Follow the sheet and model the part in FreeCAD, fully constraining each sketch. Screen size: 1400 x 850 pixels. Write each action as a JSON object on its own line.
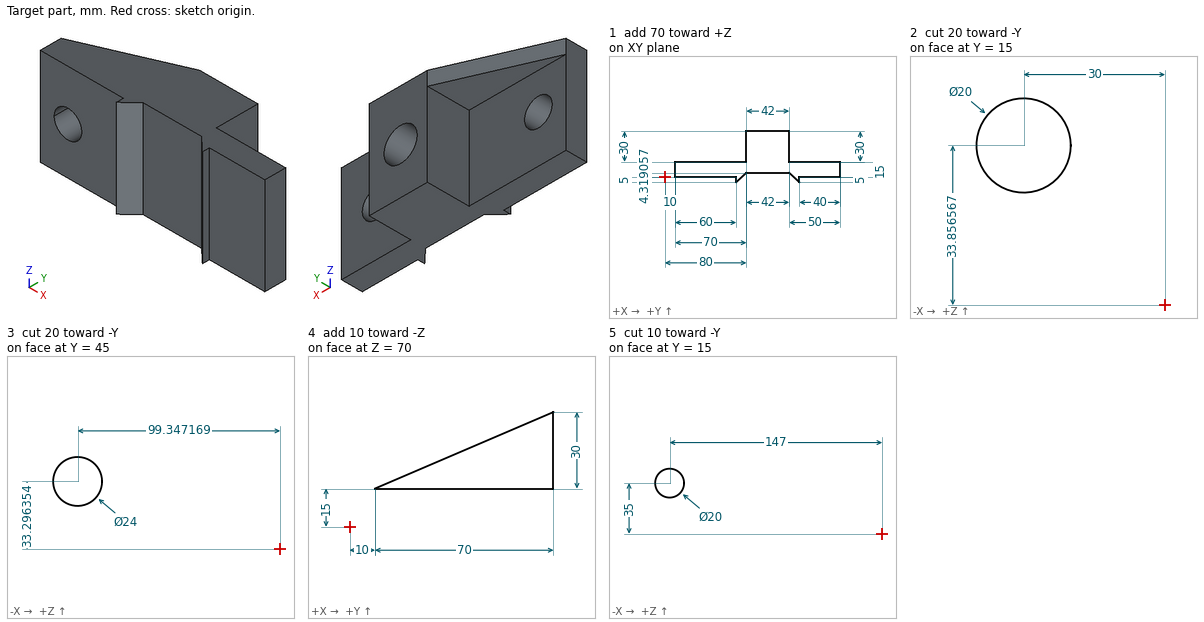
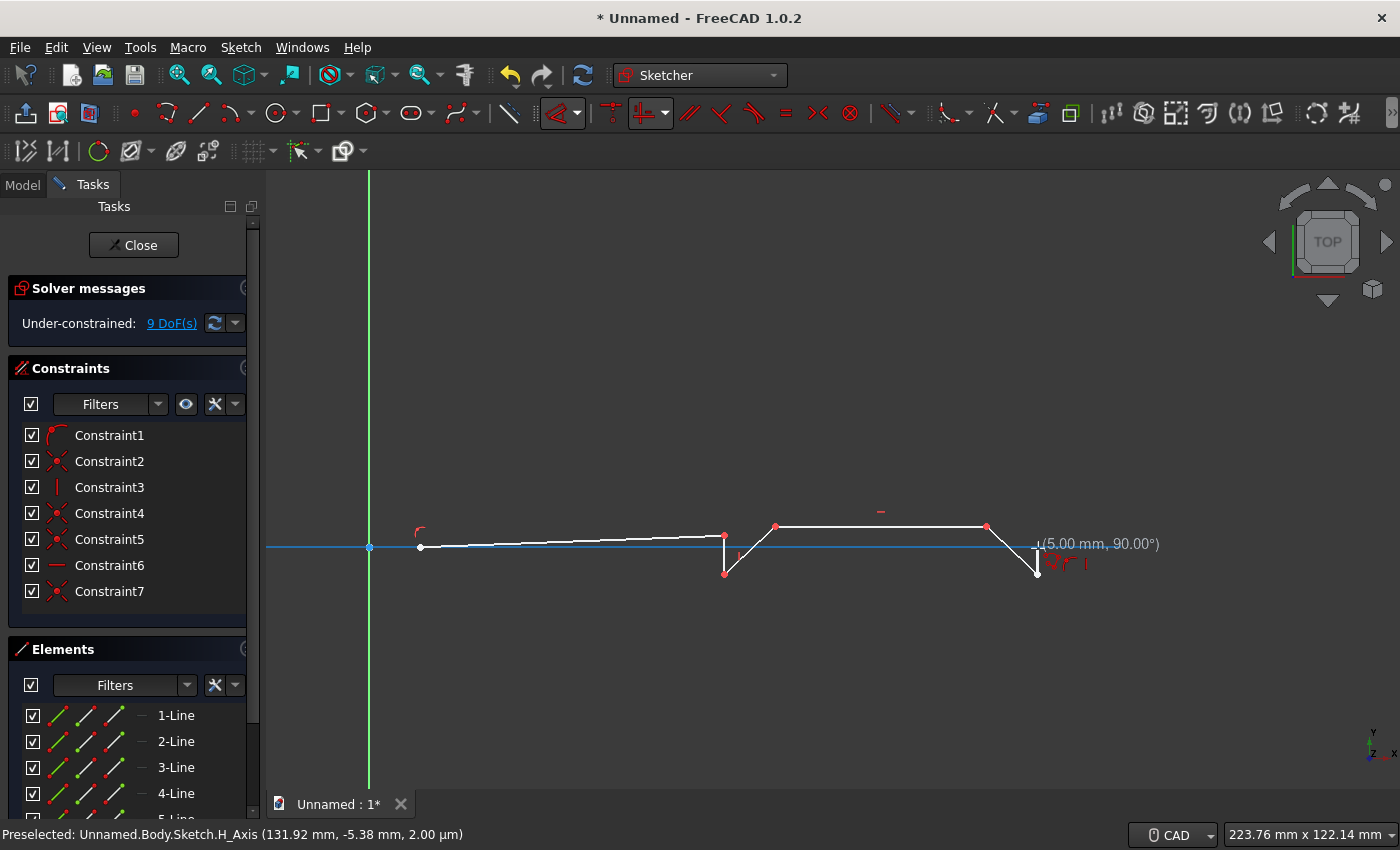
{"action": "left_click", "coordinate": [1038, 547]}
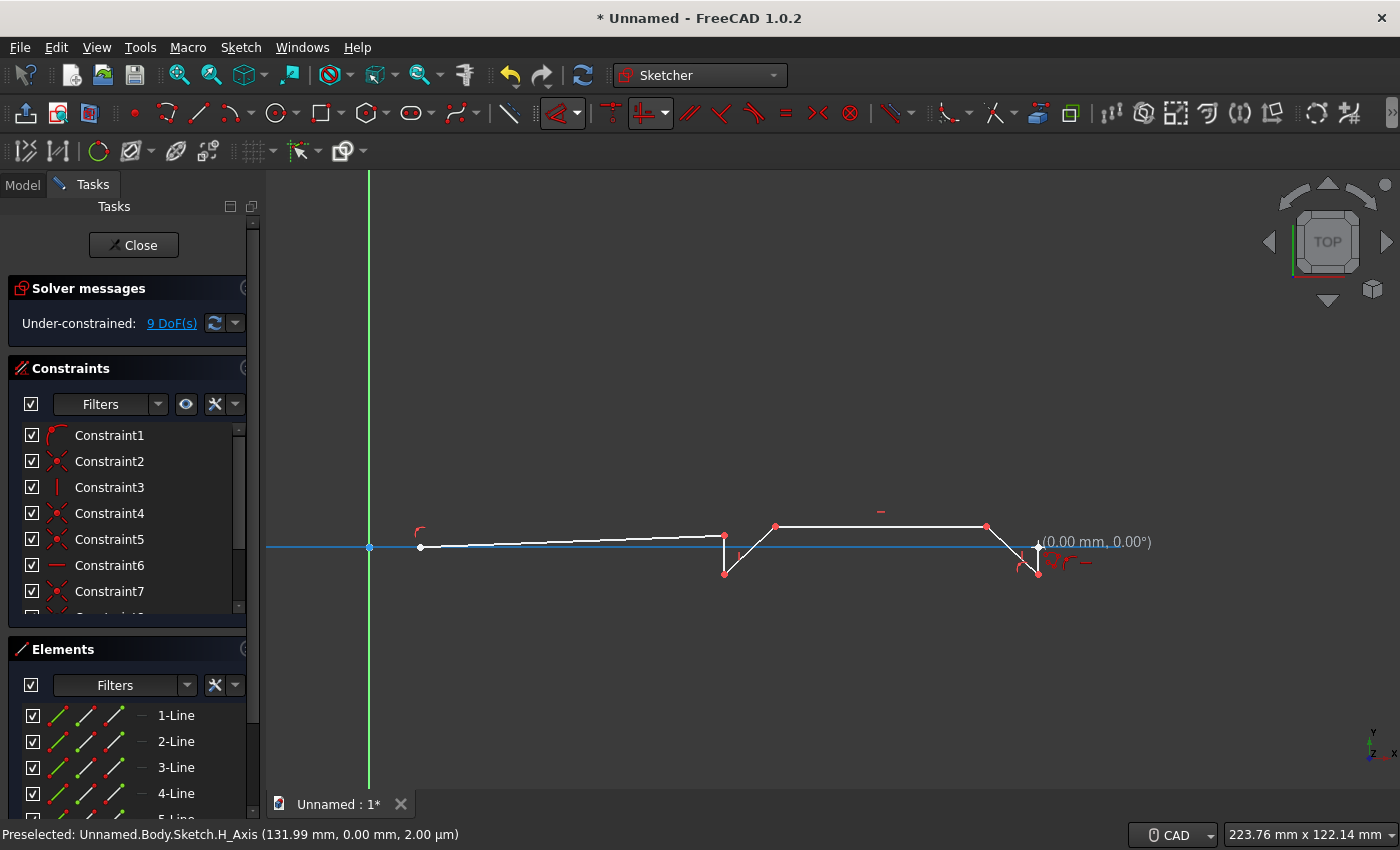
{"action": "scroll", "coordinate": [582, 631], "scroll_direction": "down", "scroll_amount": 1}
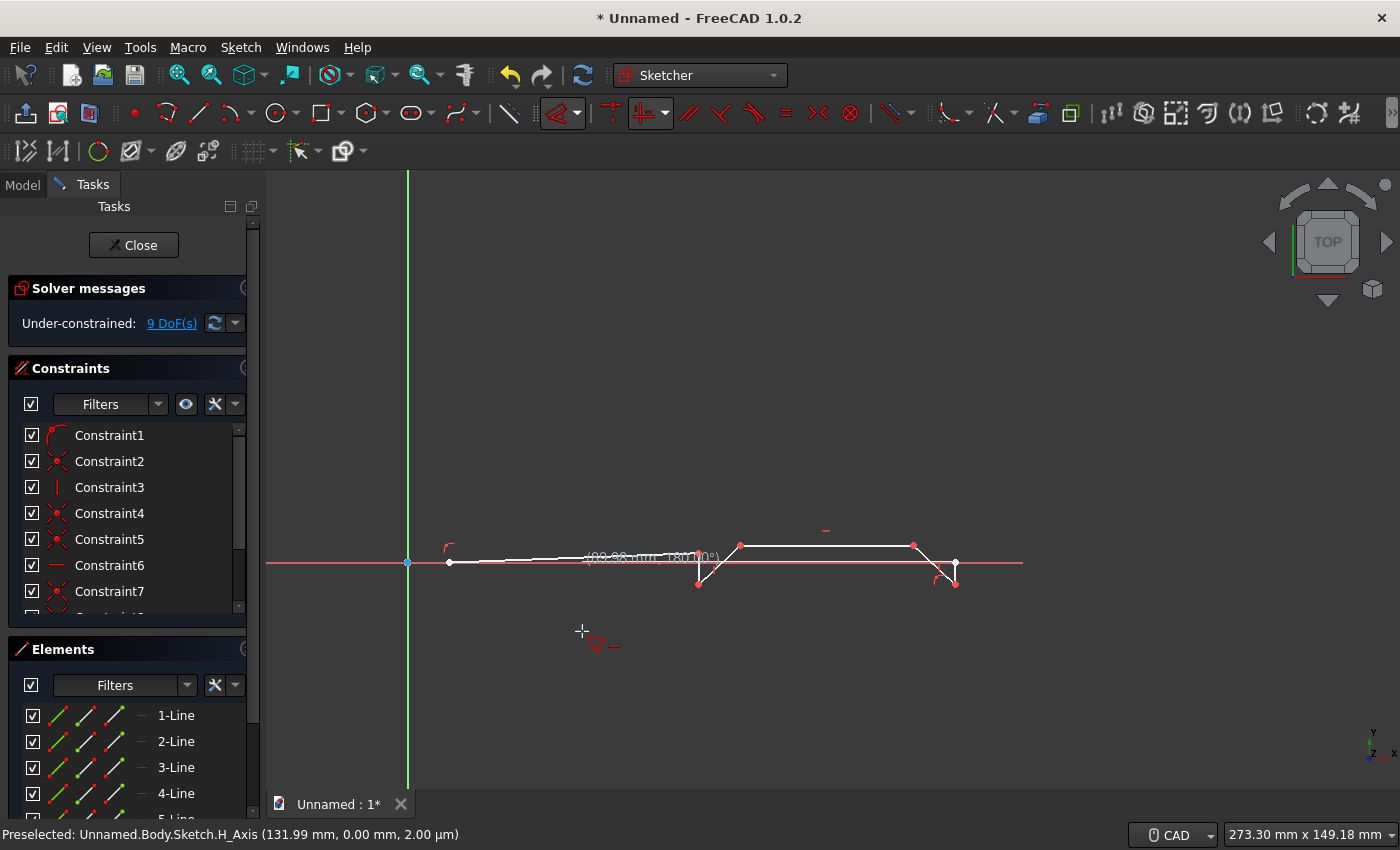
{"action": "left_click", "coordinate": [1121, 554]}
{"action": "left_click", "coordinate": [1121, 500]}
{"action": "left_click", "coordinate": [914, 500]}
{"action": "left_click", "coordinate": [914, 376]}
{"action": "left_click", "coordinate": [740, 376]}
{"action": "left_click", "coordinate": [740, 500]}
{"action": "left_click", "coordinate": [449, 500]}
{"action": "left_click", "coordinate": [449, 563]}
{"action": "key", "text": "Escape"}
{"action": "key", "text": "Escape"}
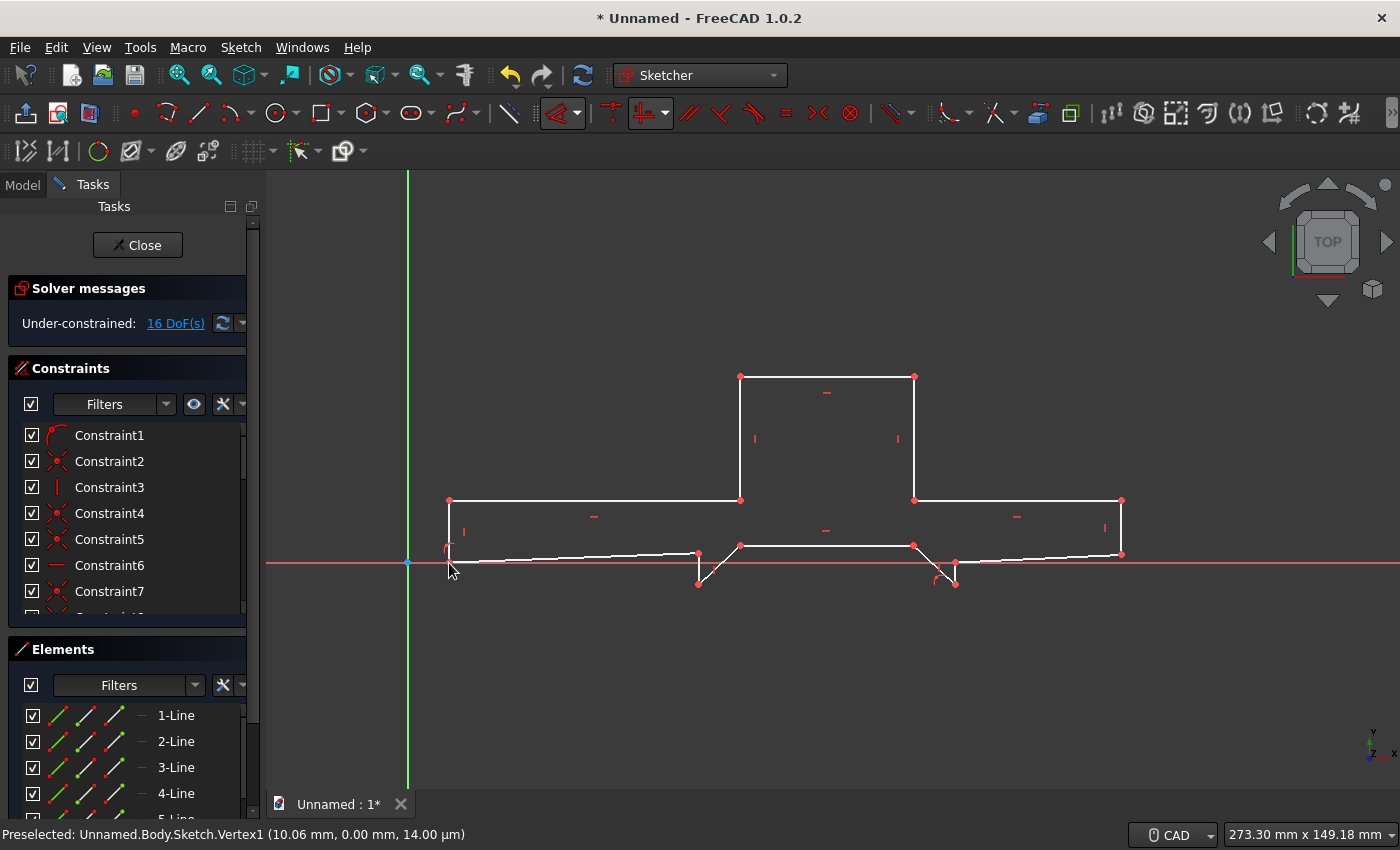
{"action": "left_click", "coordinate": [524, 560]}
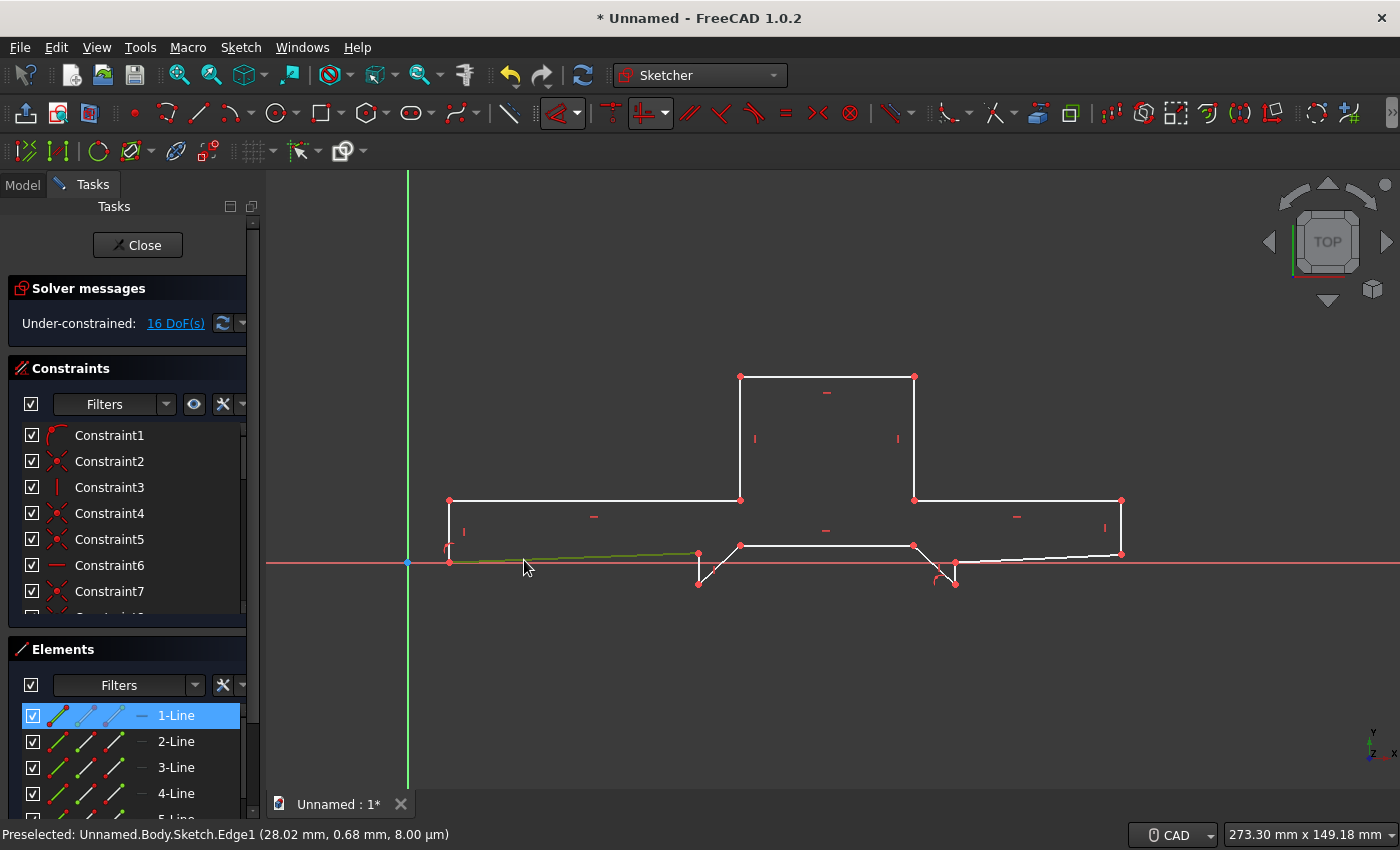
{"action": "key", "text": "h"}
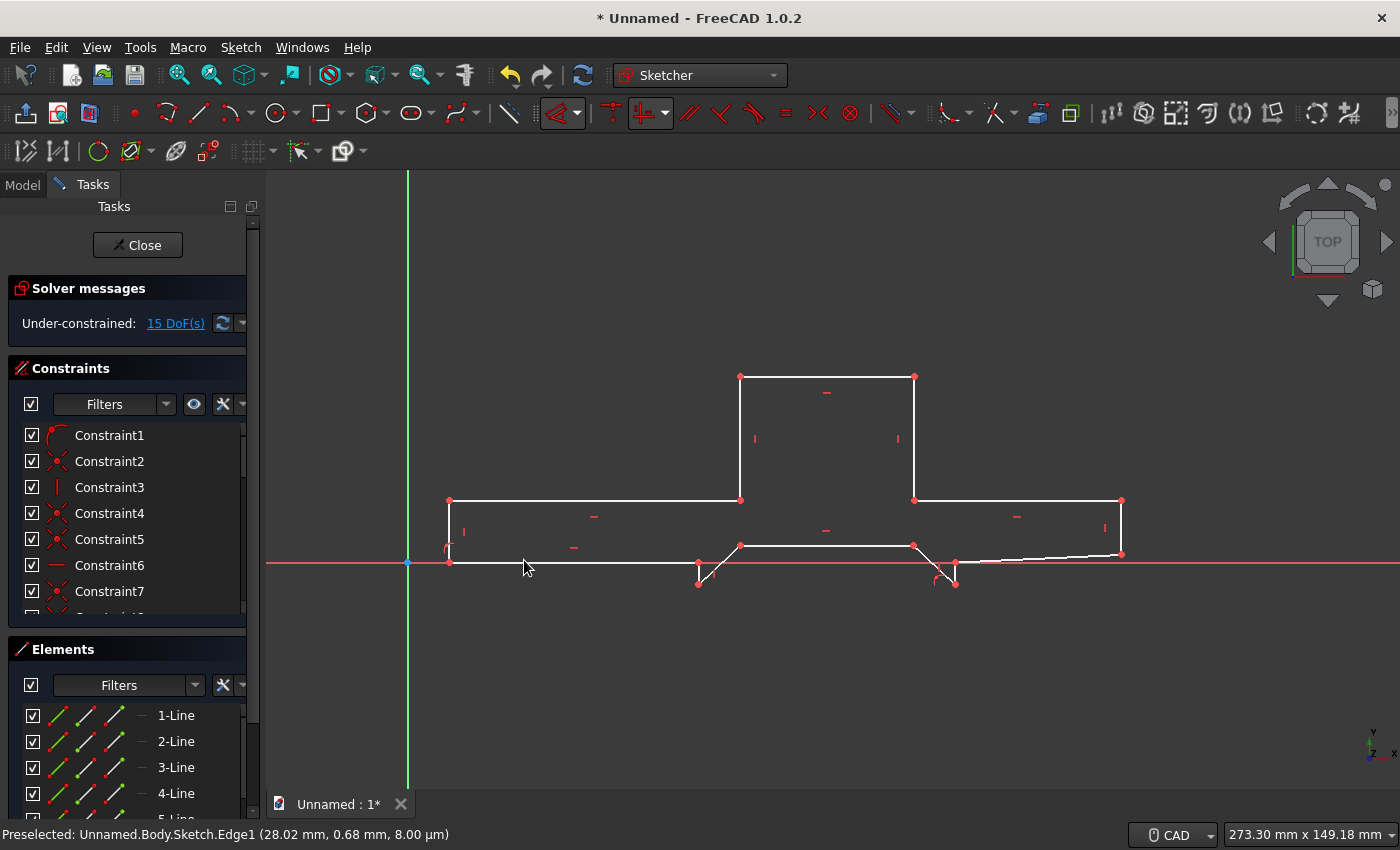
{"action": "left_click", "coordinate": [1005, 560]}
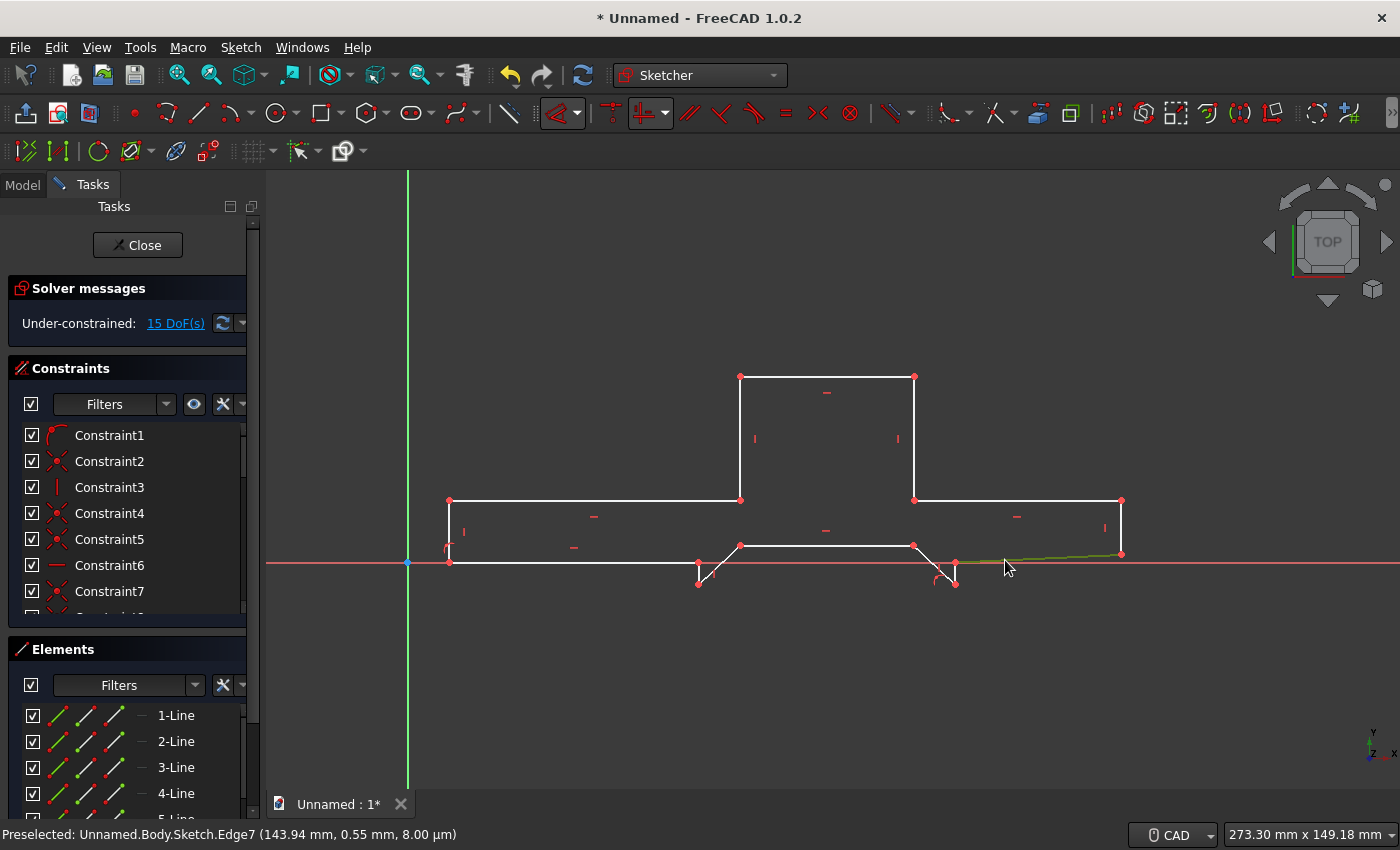
{"action": "left_click", "coordinate": [668, 114]}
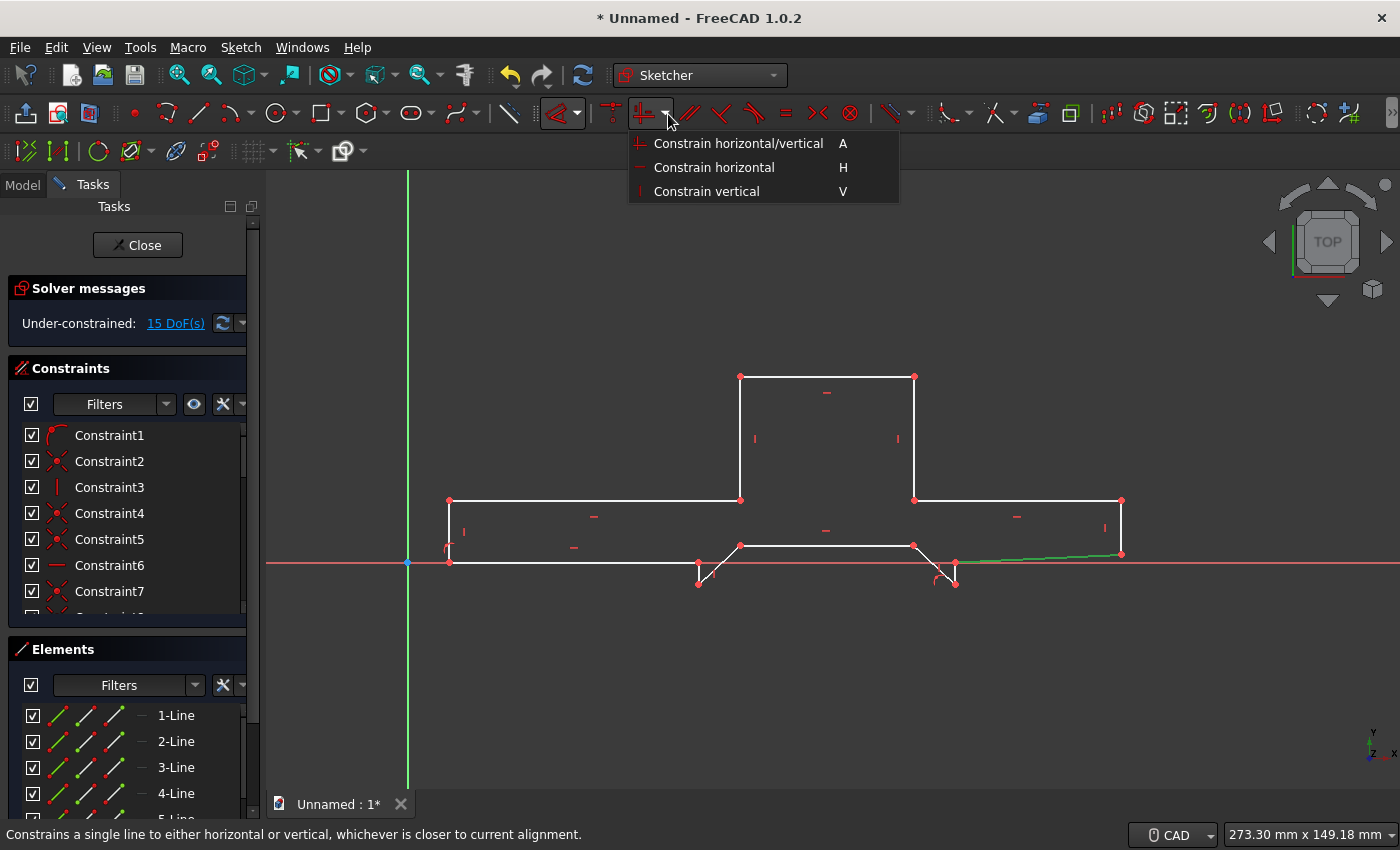
{"action": "left_click", "coordinate": [764, 167]}